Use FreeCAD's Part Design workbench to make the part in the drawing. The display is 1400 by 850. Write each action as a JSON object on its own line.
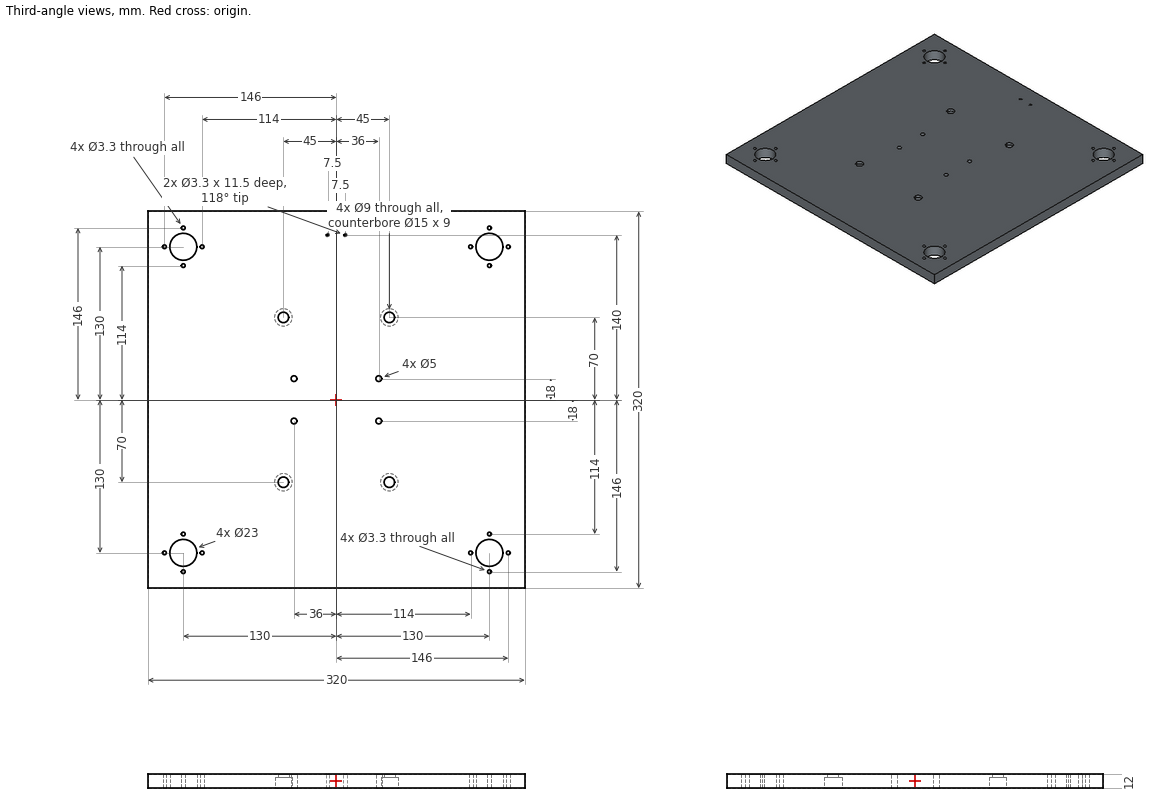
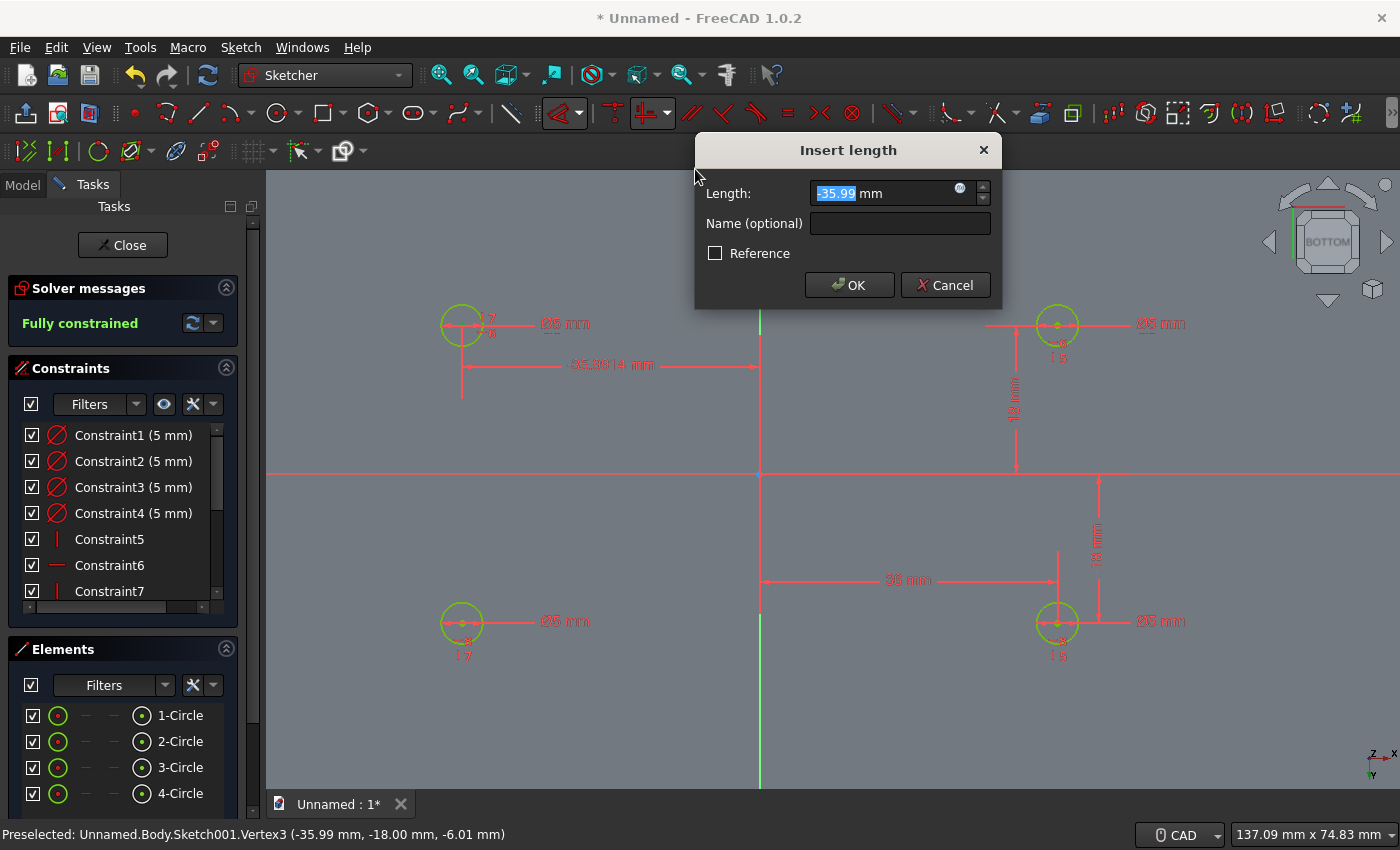
{"action": "type", "text": "-36"}
{"action": "key", "text": "Return"}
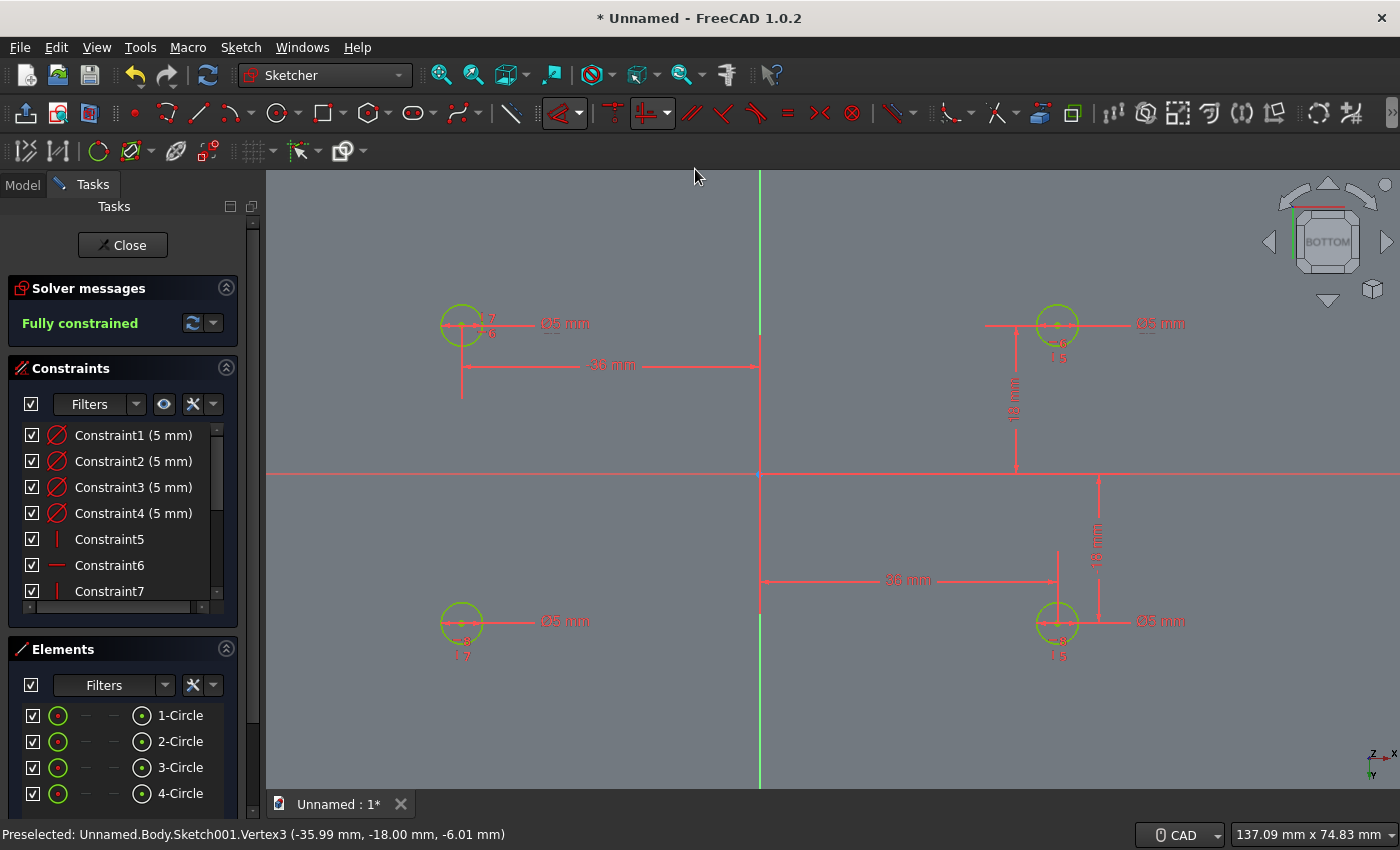
{"action": "left_click", "coordinate": [123, 245]}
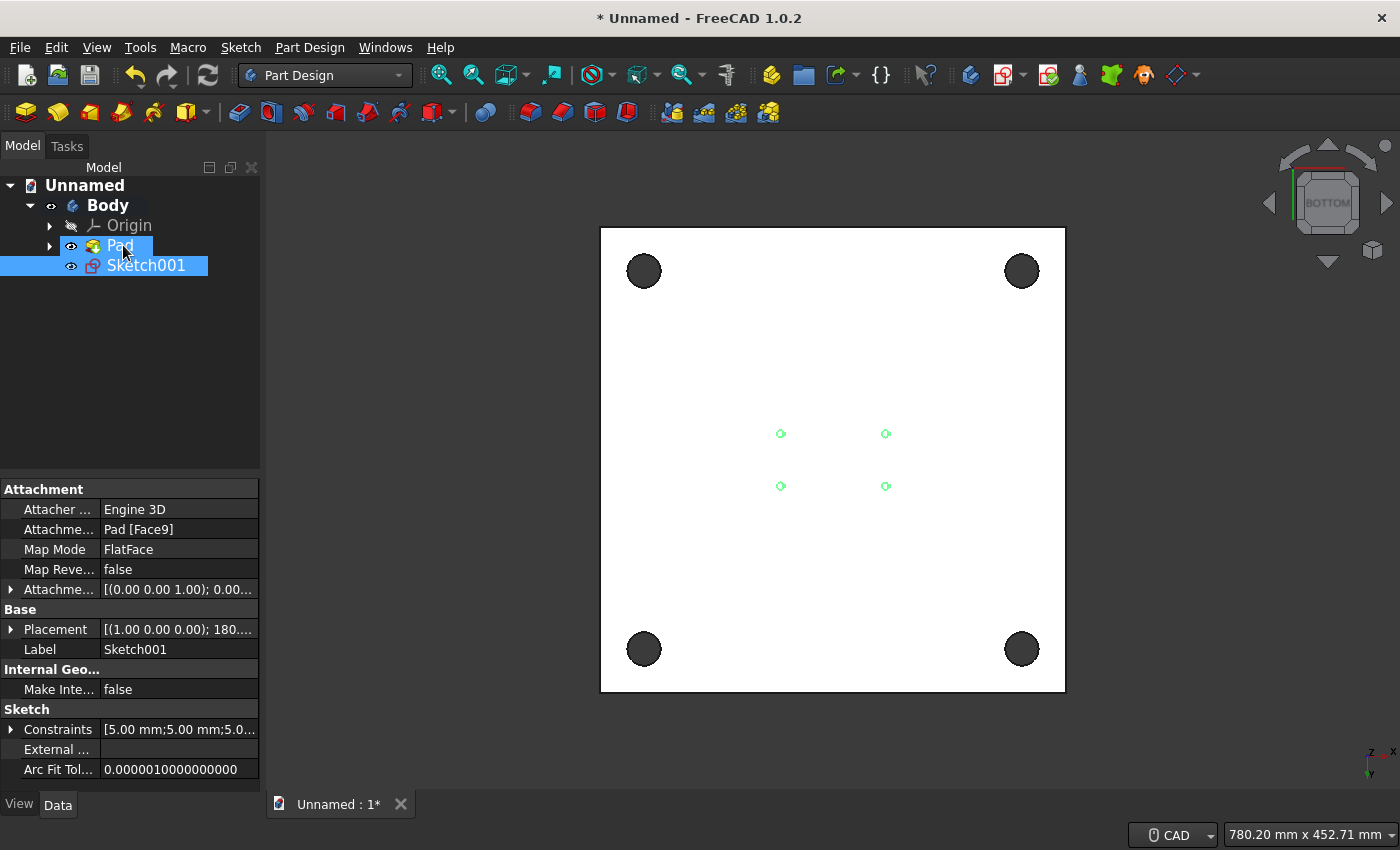
{"action": "left_click", "coordinate": [240, 112]}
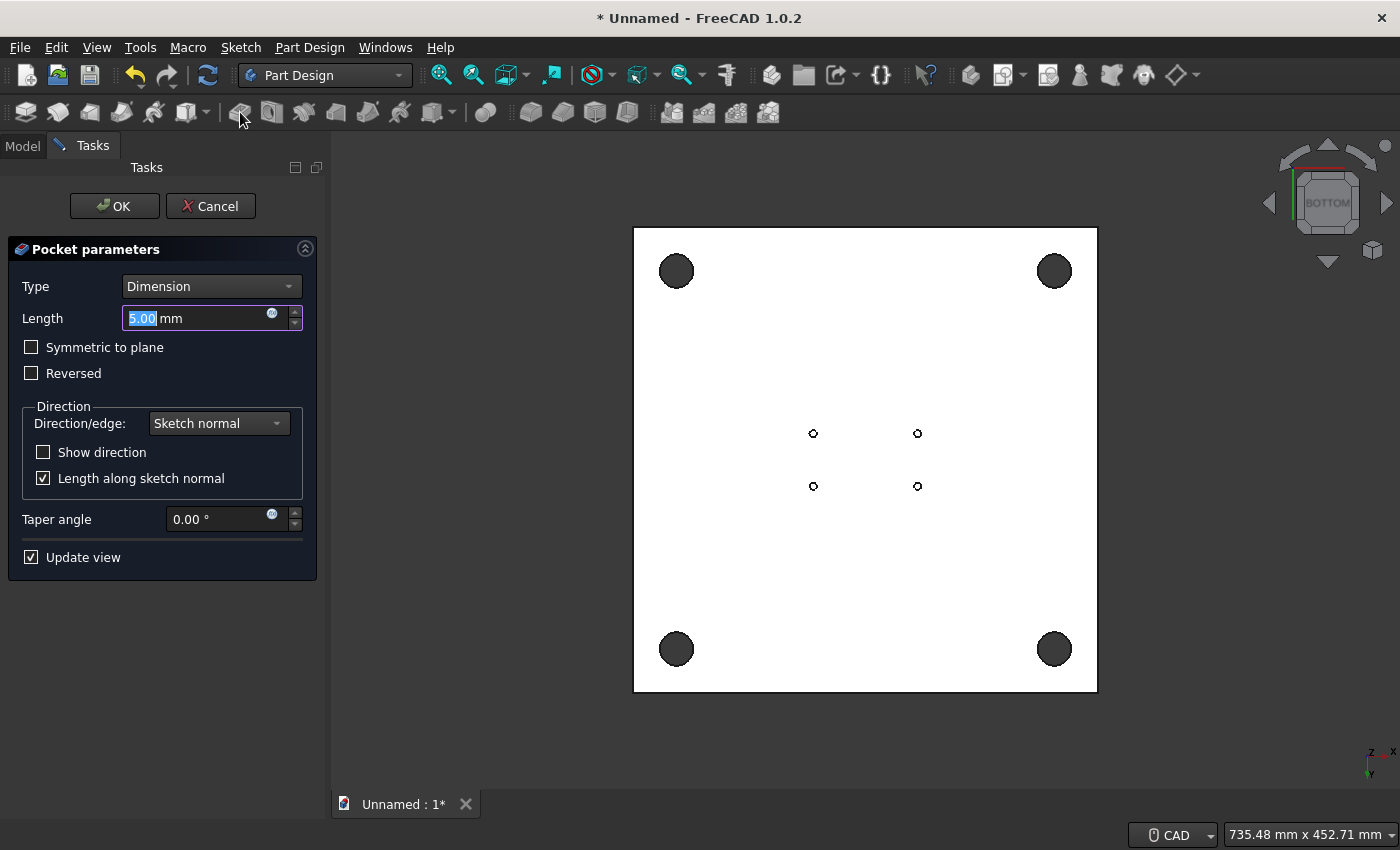
{"action": "left_click", "coordinate": [212, 286]}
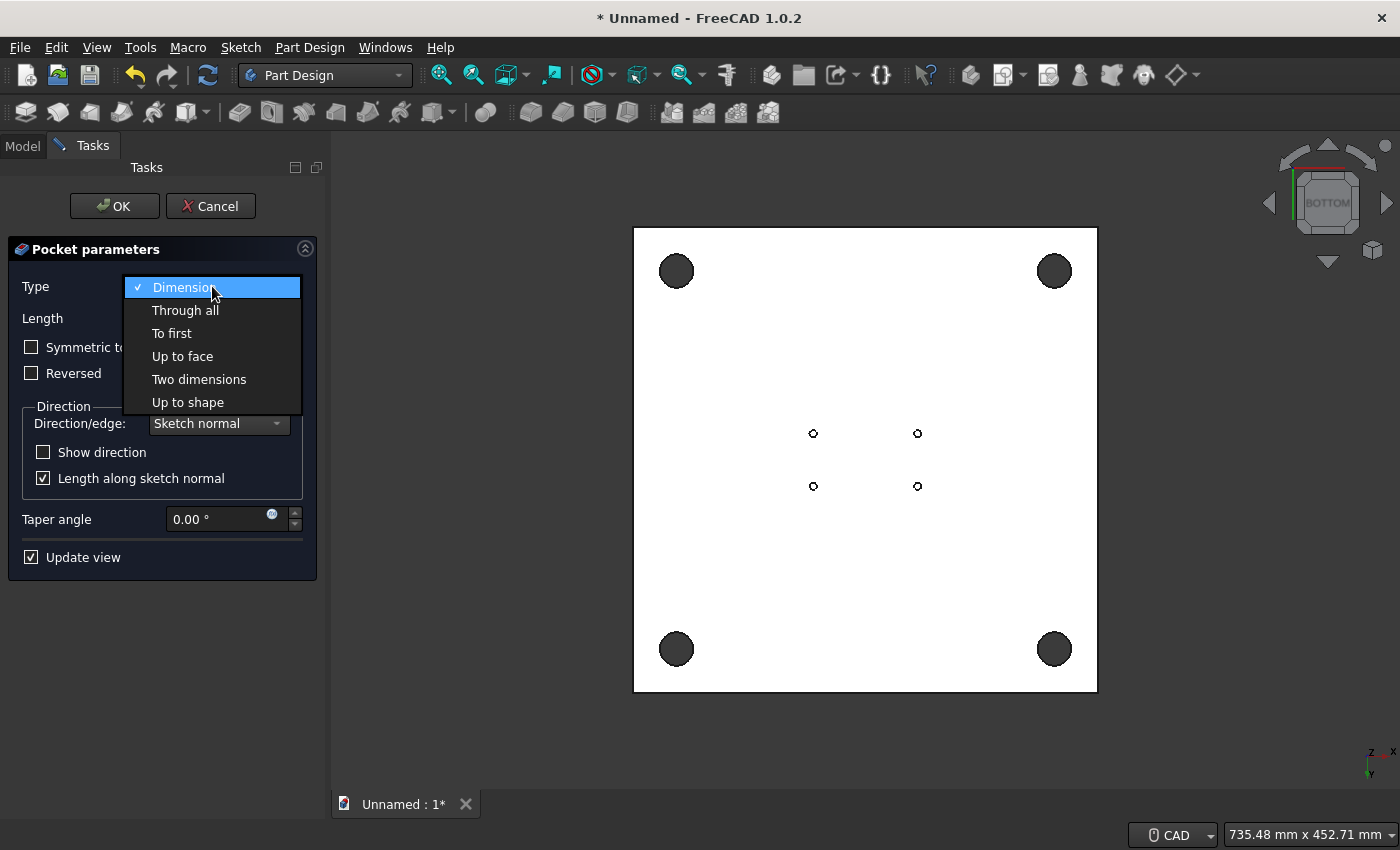
{"action": "left_click", "coordinate": [212, 310]}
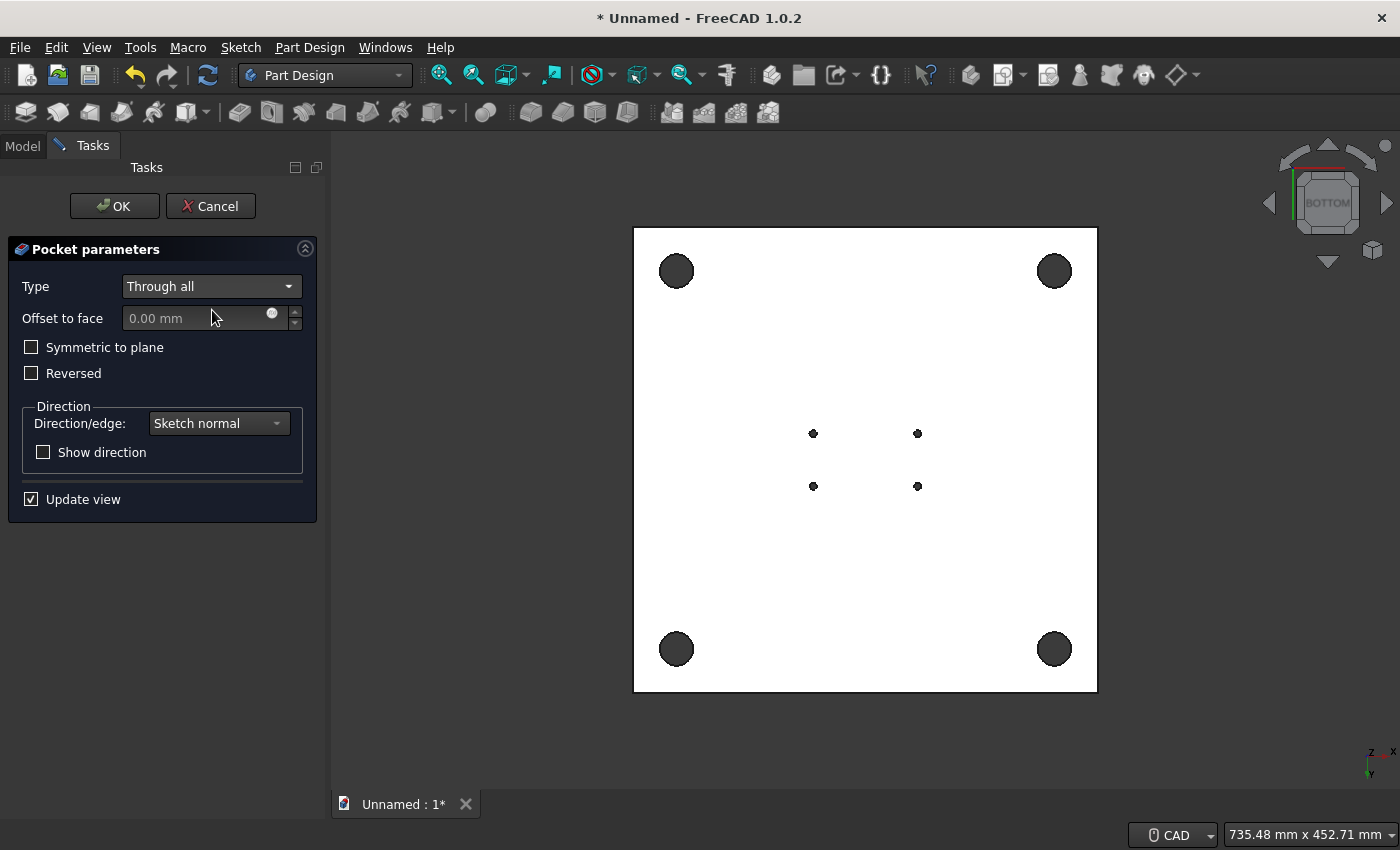
{"action": "left_click", "coordinate": [115, 206]}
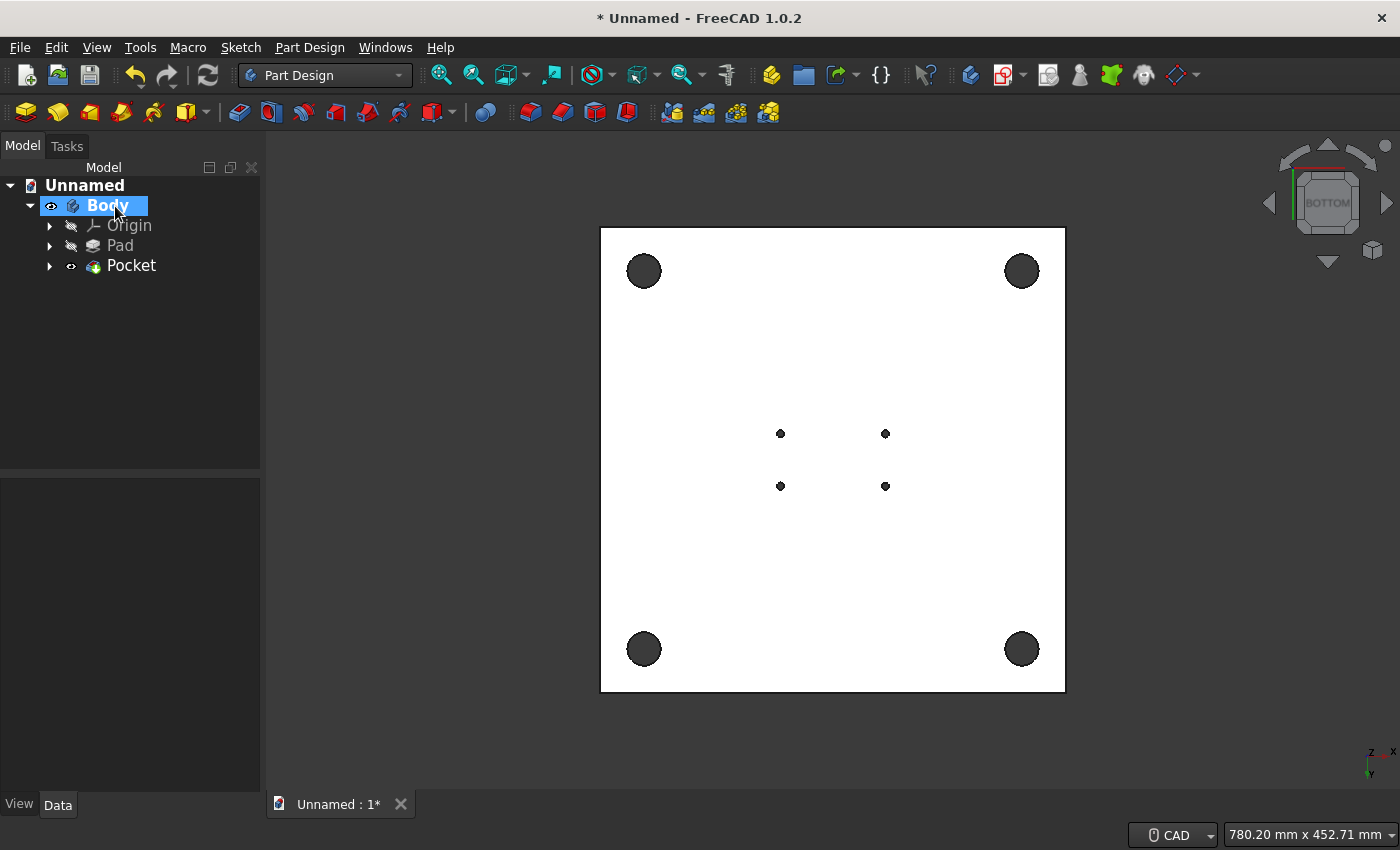
{"action": "left_click", "coordinate": [899, 592]}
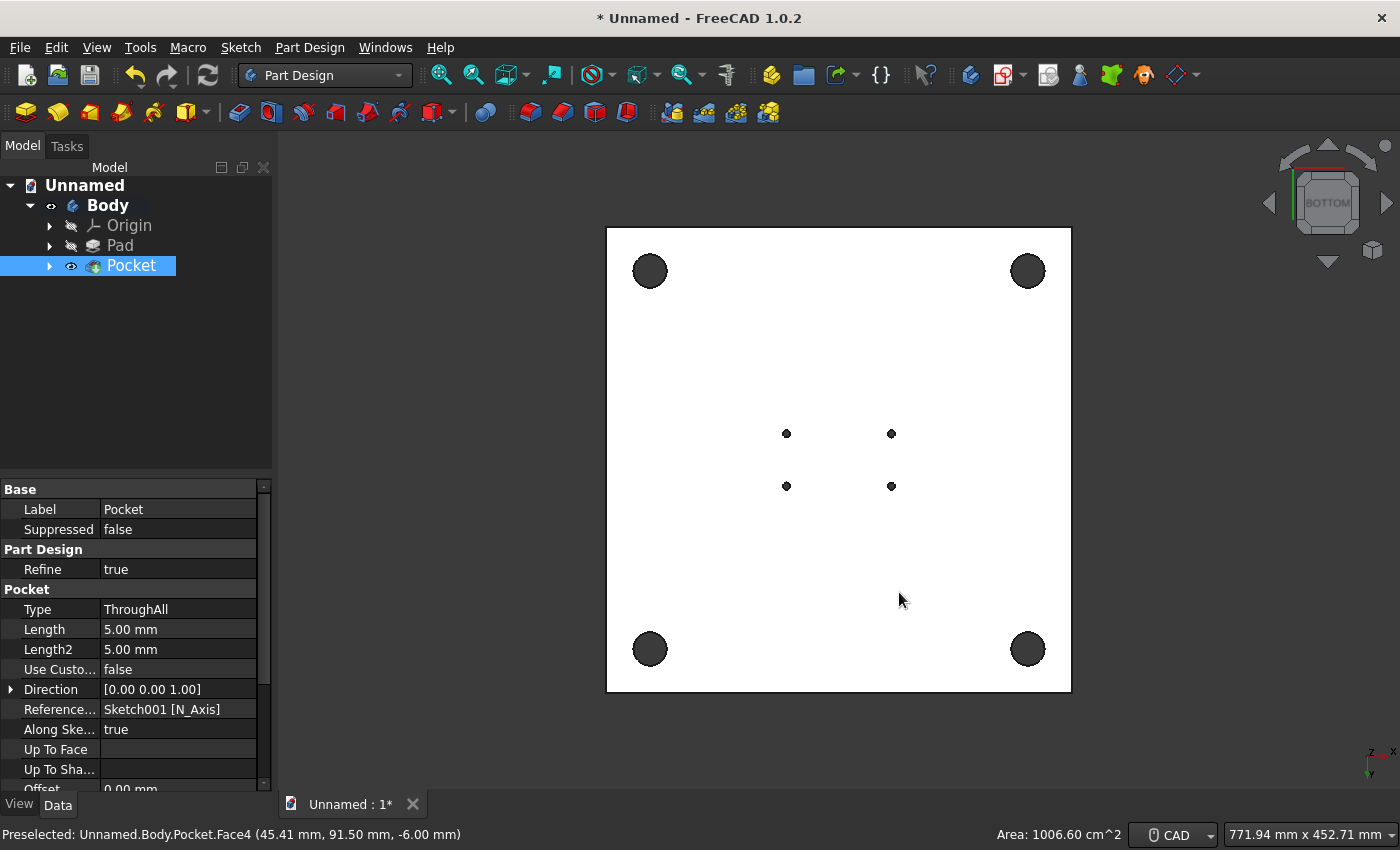
{"action": "left_click", "coordinate": [1004, 76]}